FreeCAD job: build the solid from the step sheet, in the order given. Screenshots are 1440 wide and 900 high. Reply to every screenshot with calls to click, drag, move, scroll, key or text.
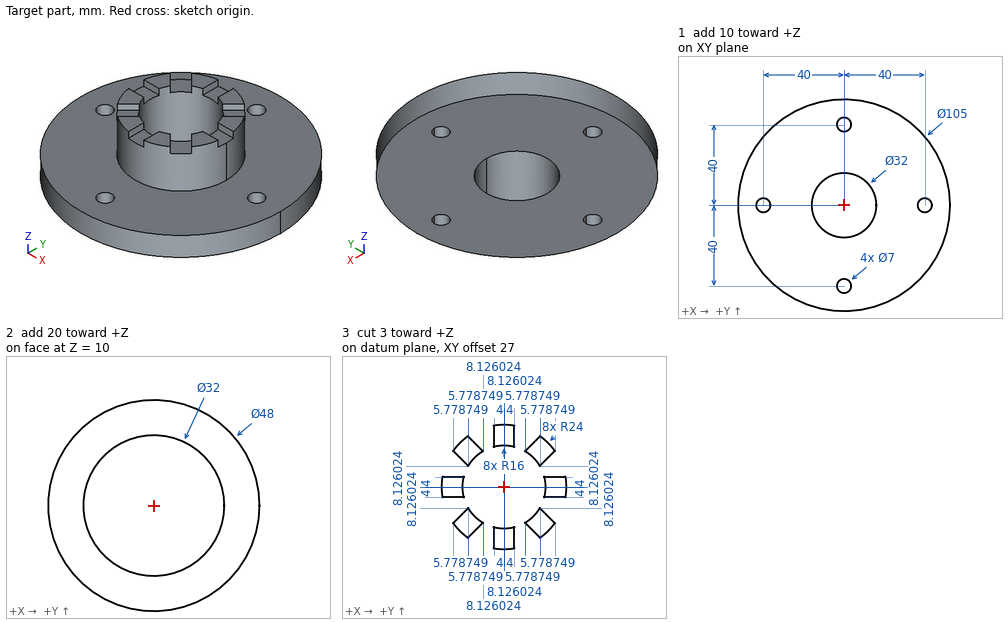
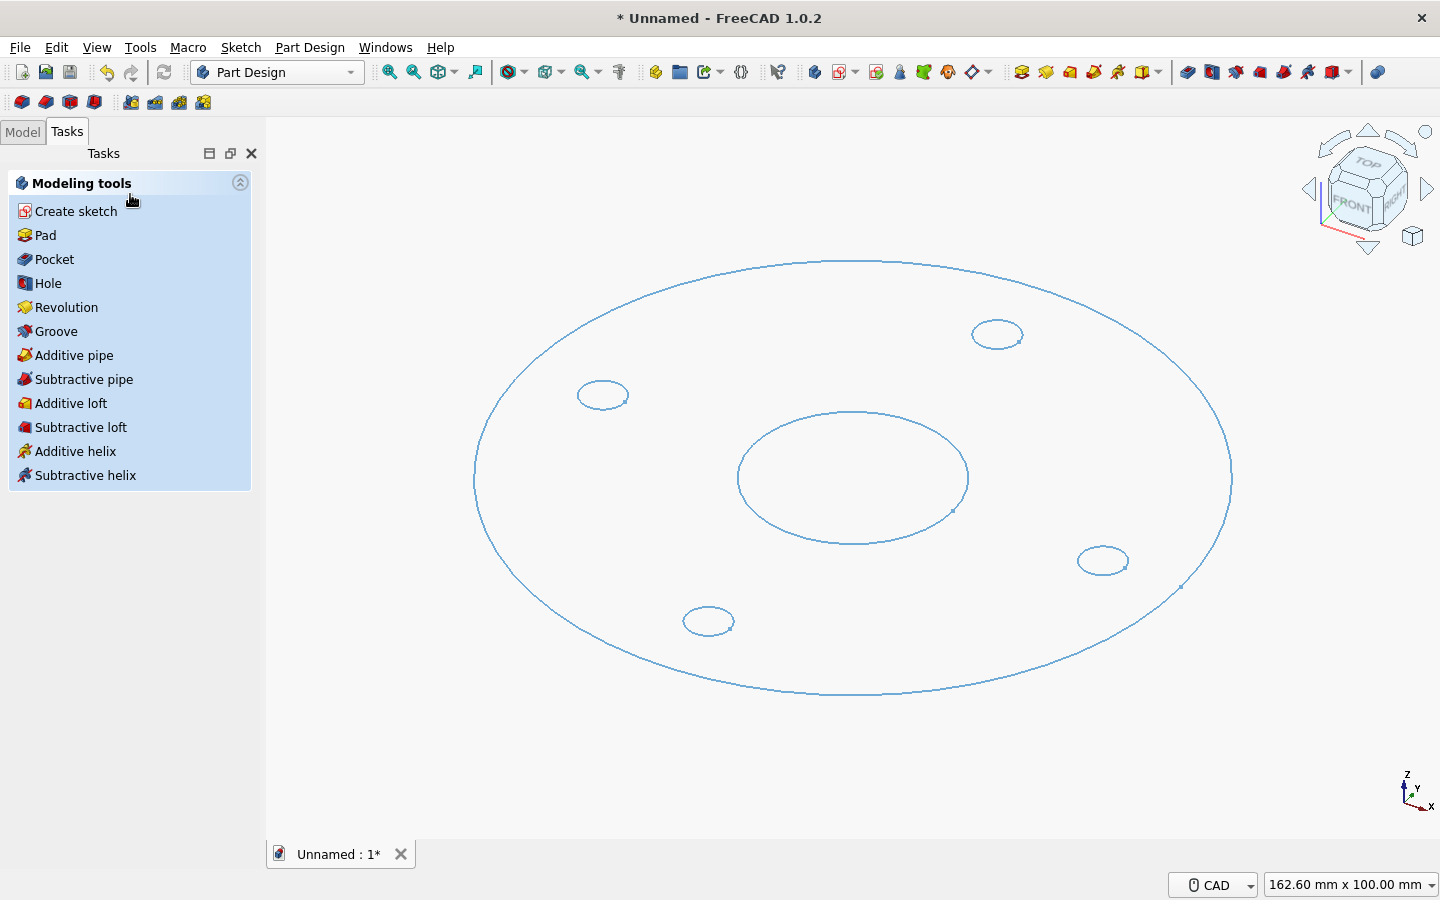
click(1022, 72)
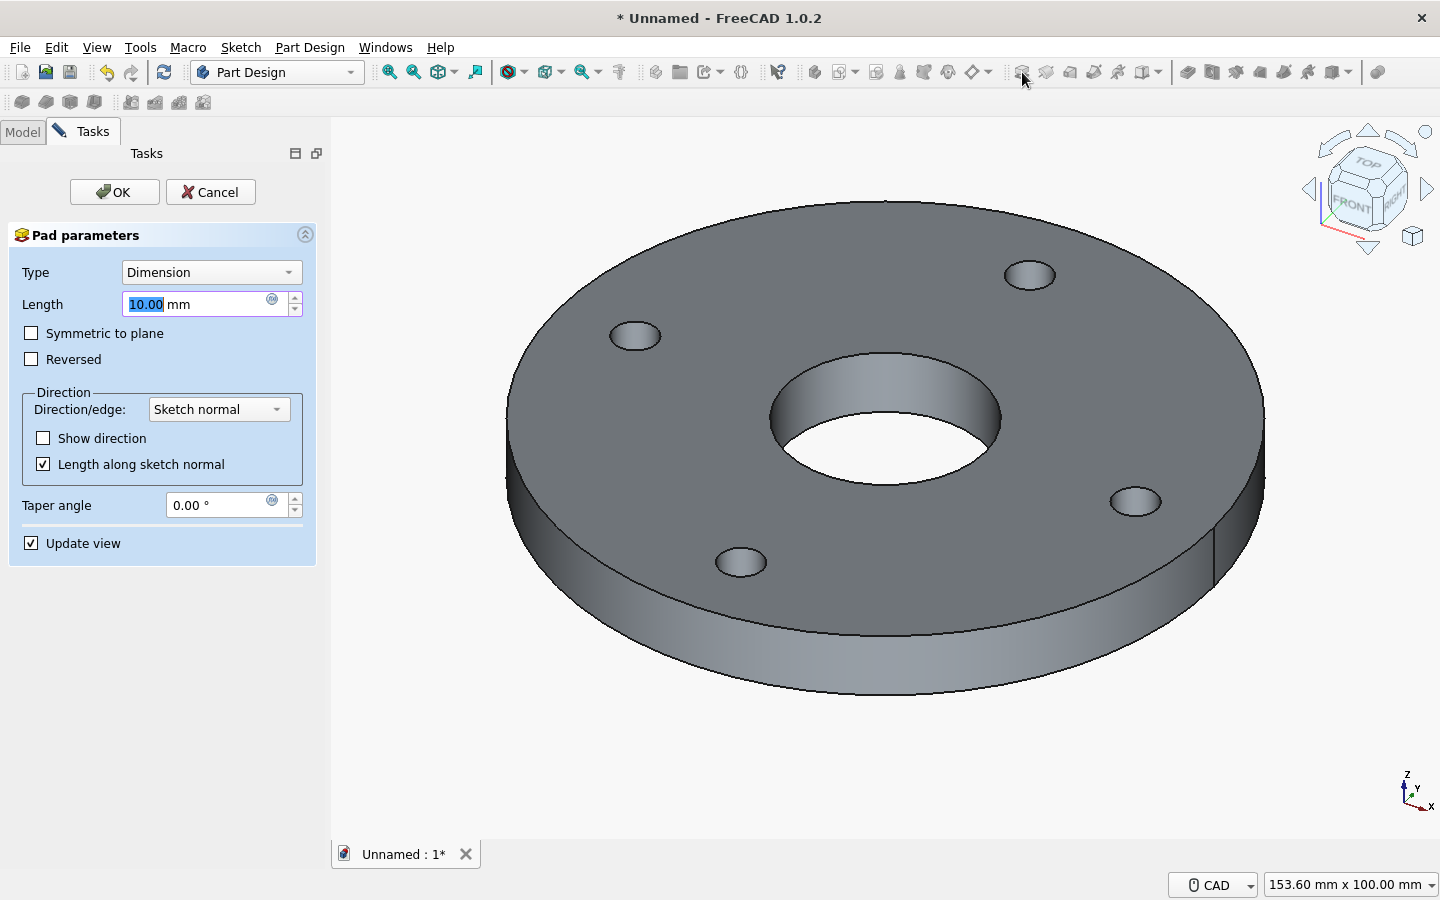
text(10)
key(Tab)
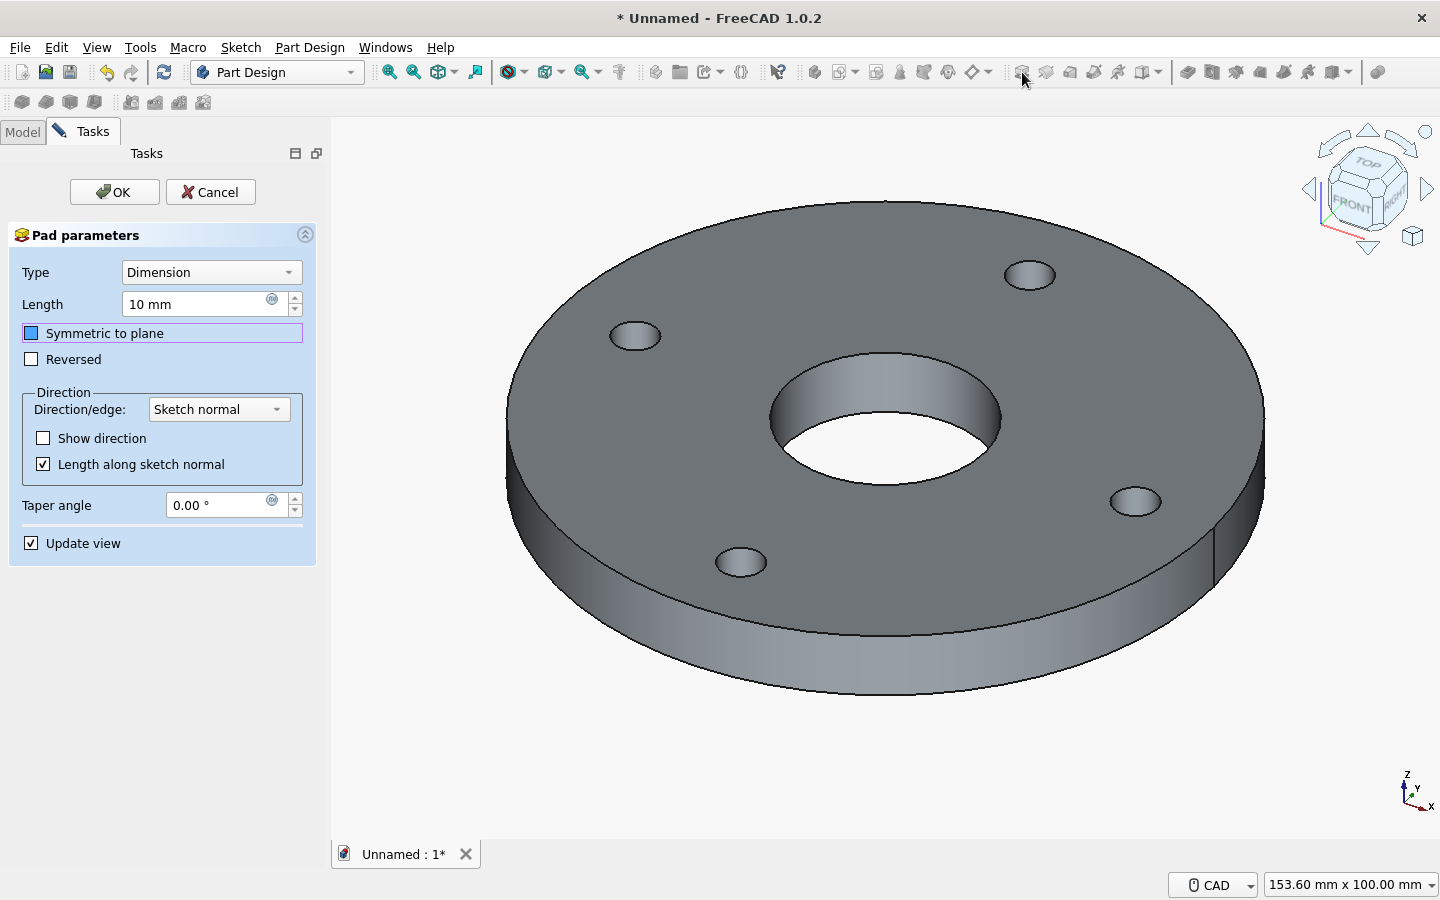
click(115, 192)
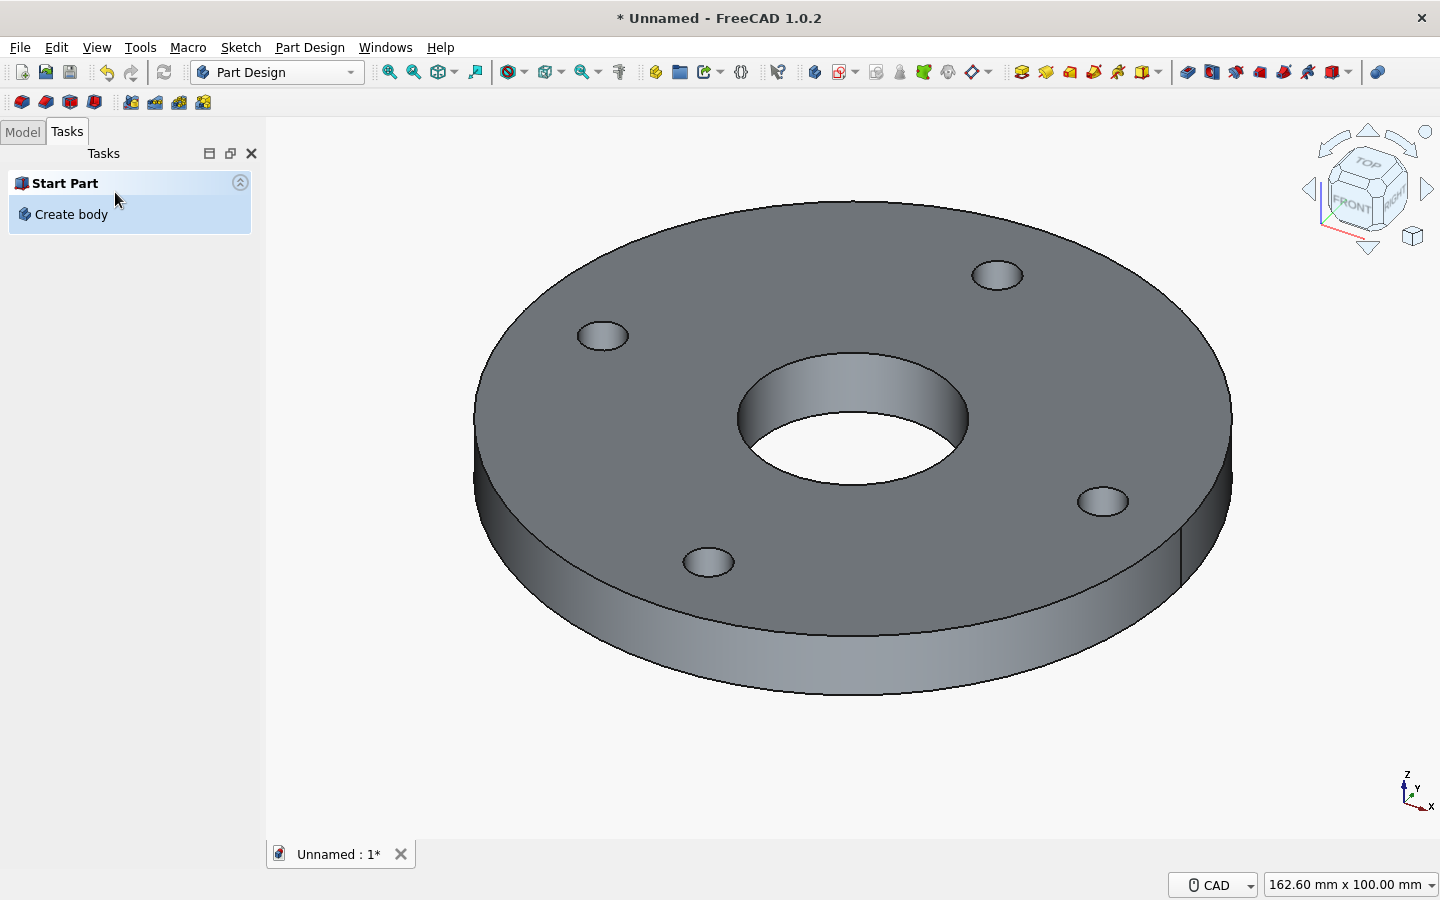
click(1095, 426)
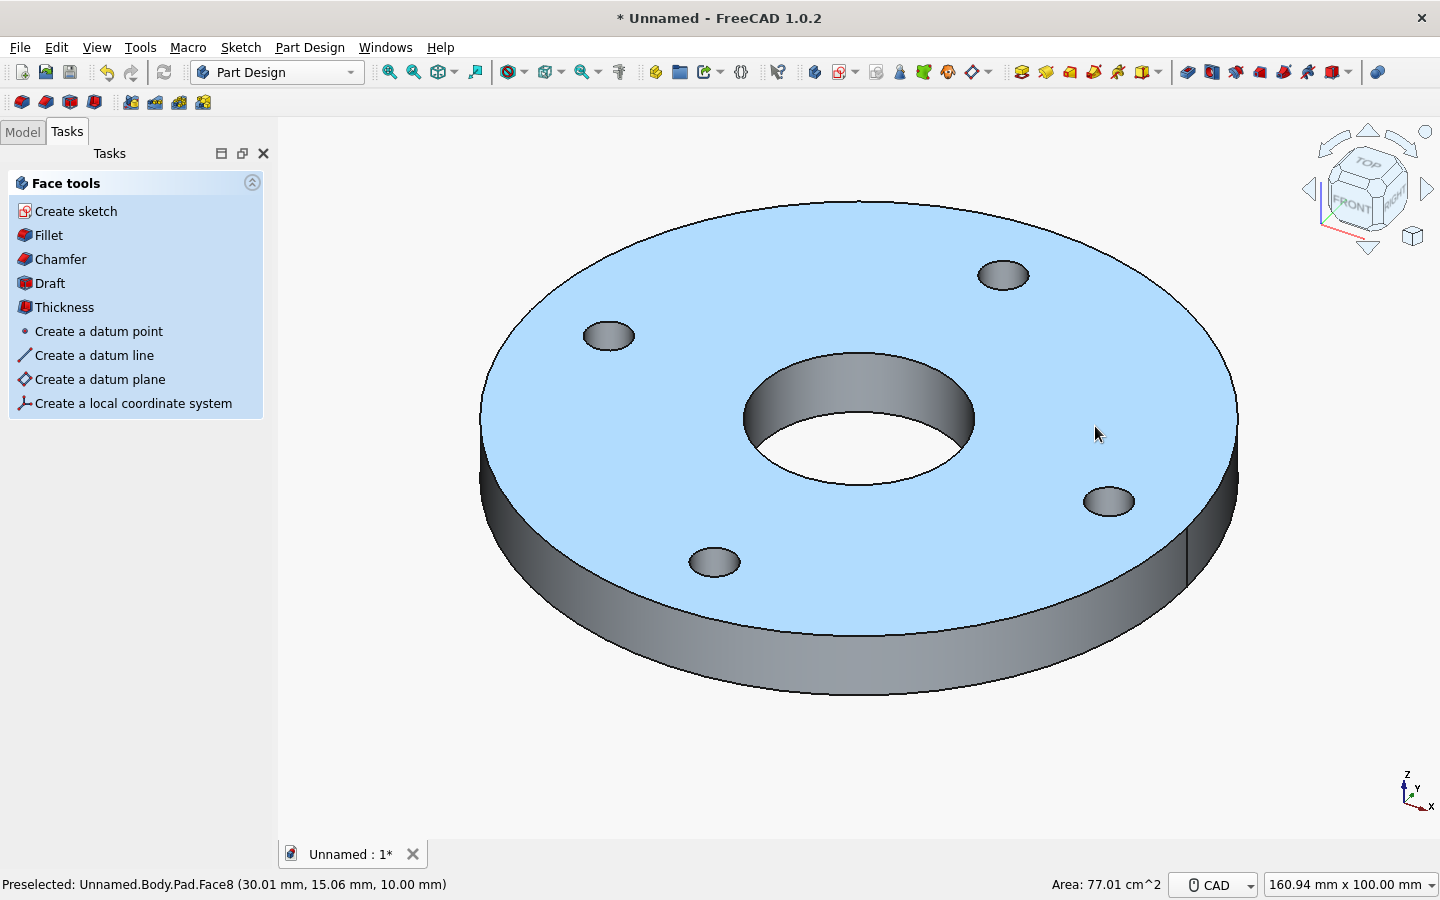
click(840, 72)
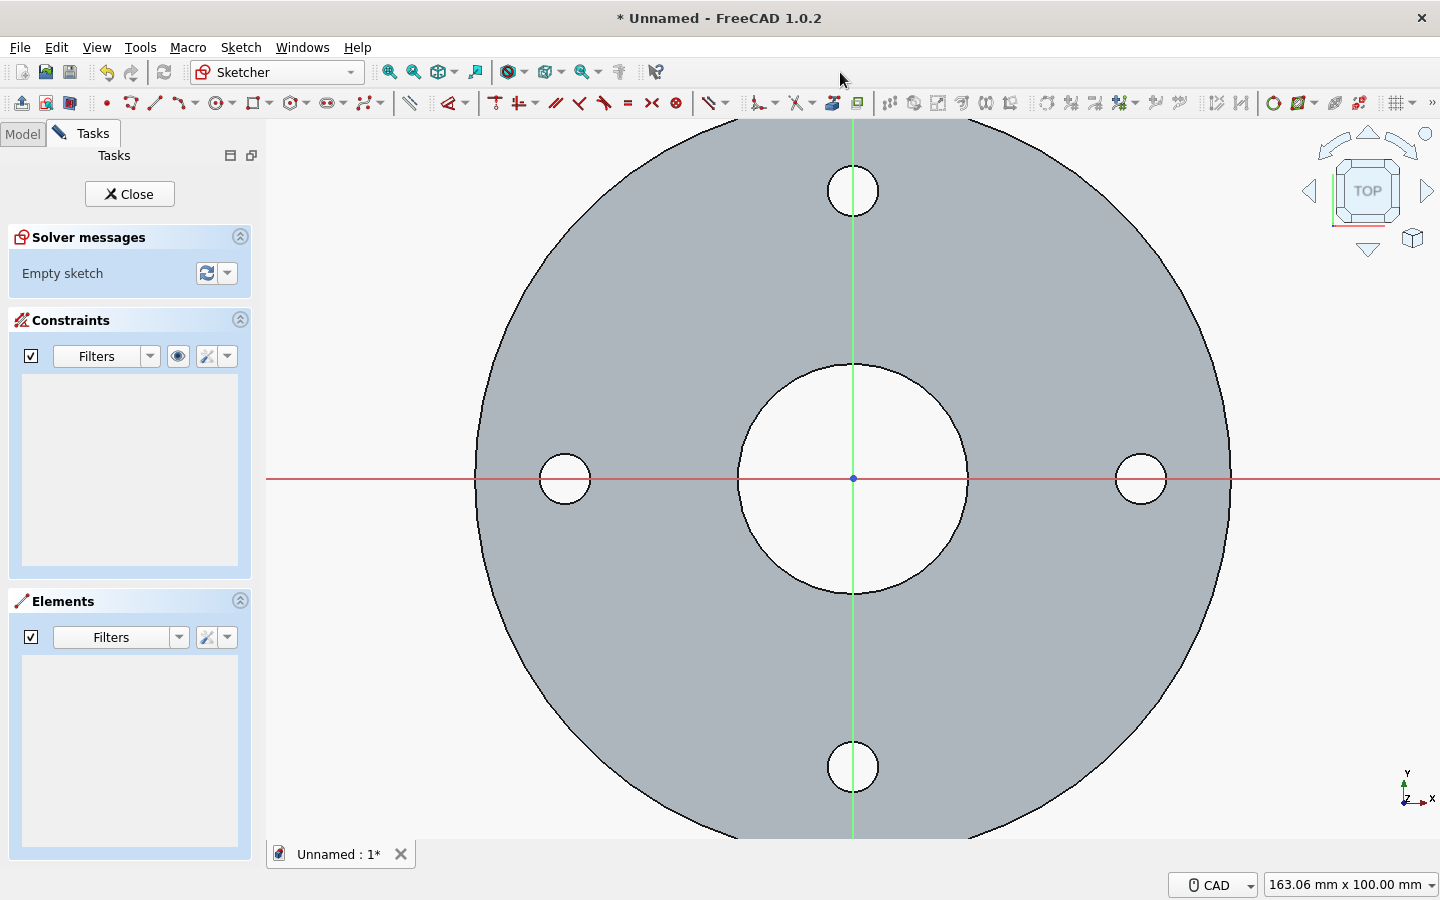
scroll(992, 479, up, 2)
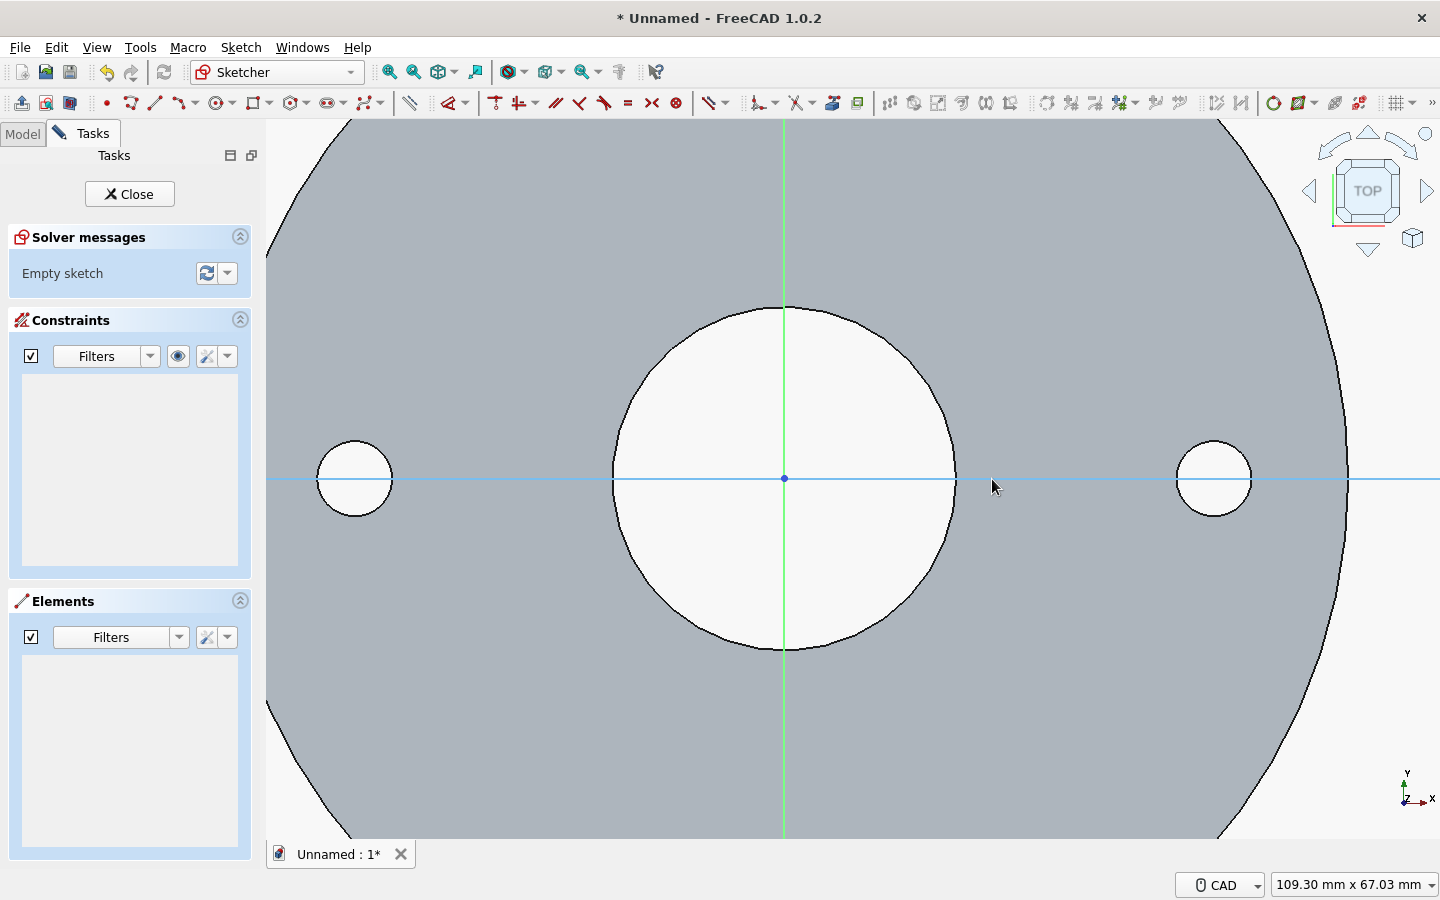
click(216, 104)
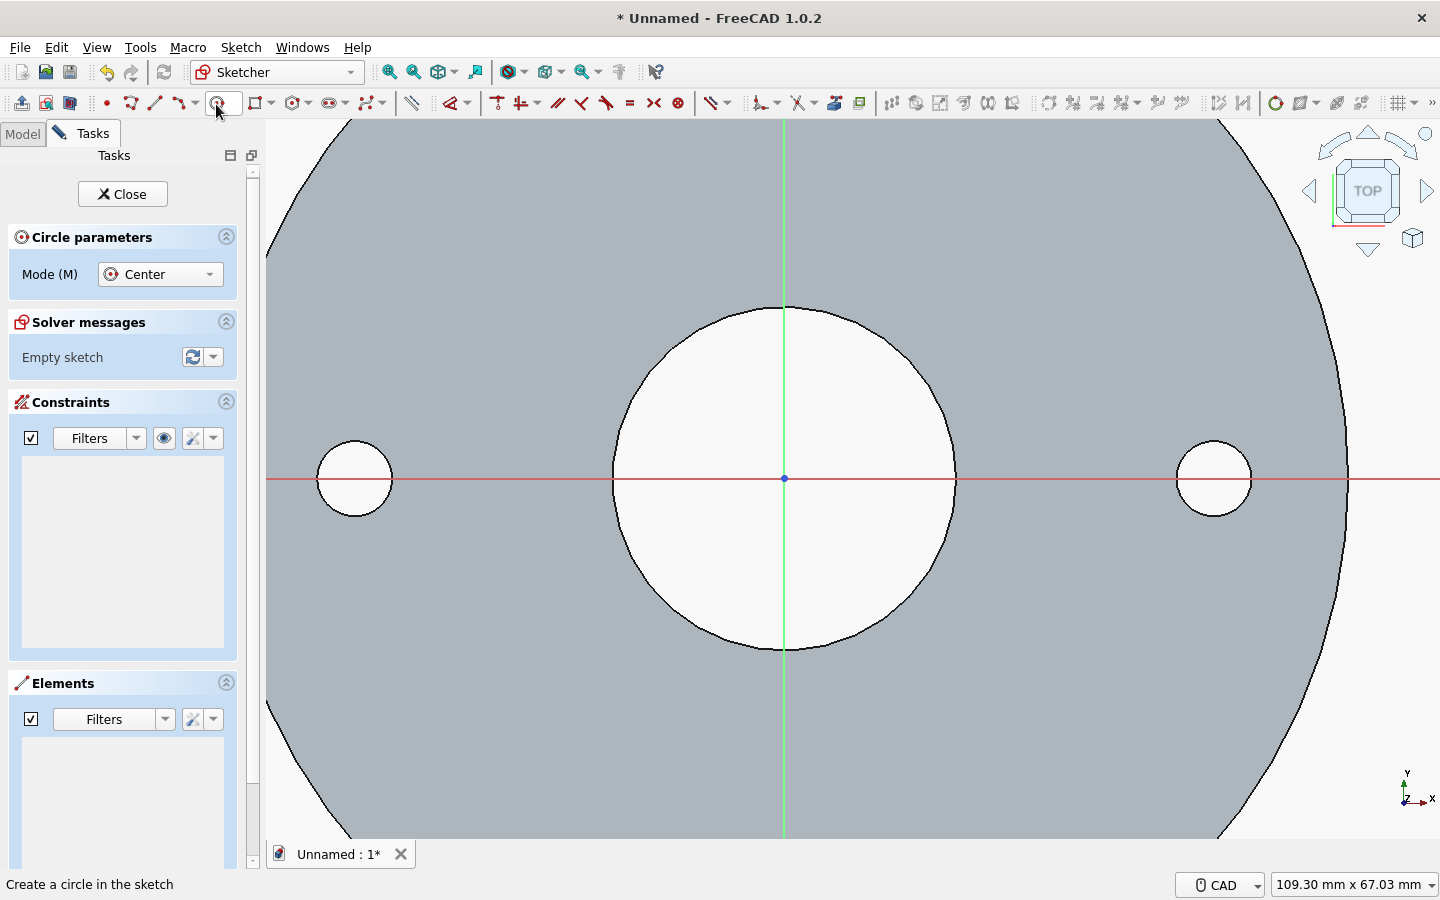
click(784, 479)
move(967, 296)